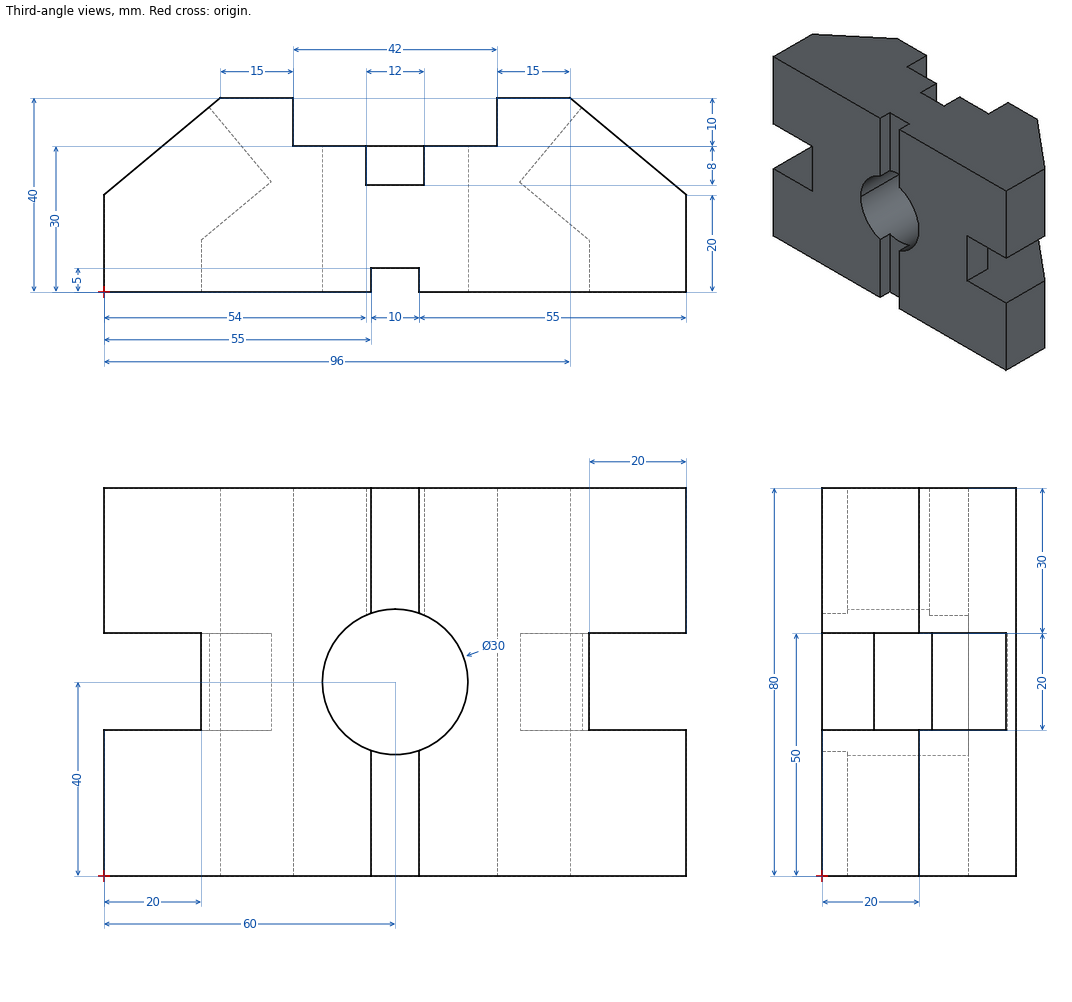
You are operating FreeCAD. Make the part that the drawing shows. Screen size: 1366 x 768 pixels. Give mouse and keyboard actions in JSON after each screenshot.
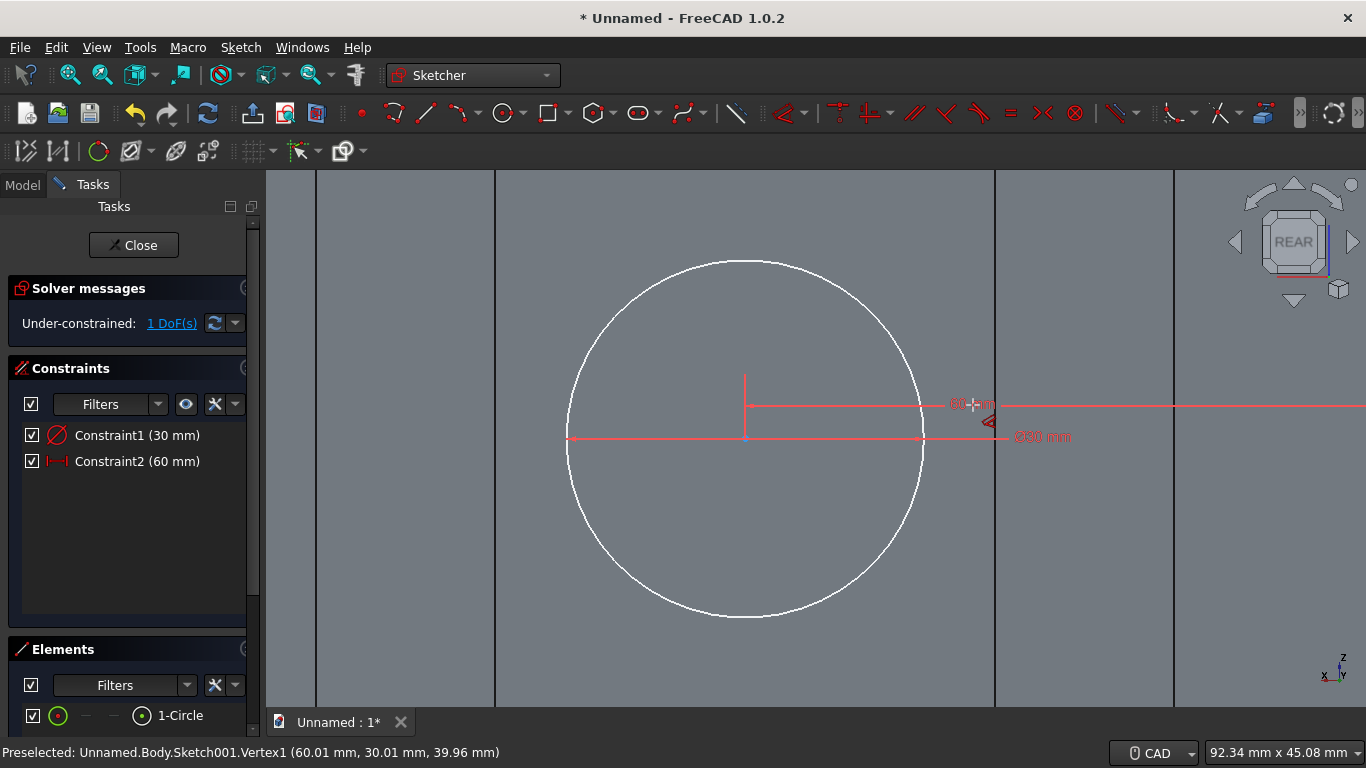
{"action": "left_click", "coordinate": [745, 439]}
{"action": "left_click", "coordinate": [711, 559]}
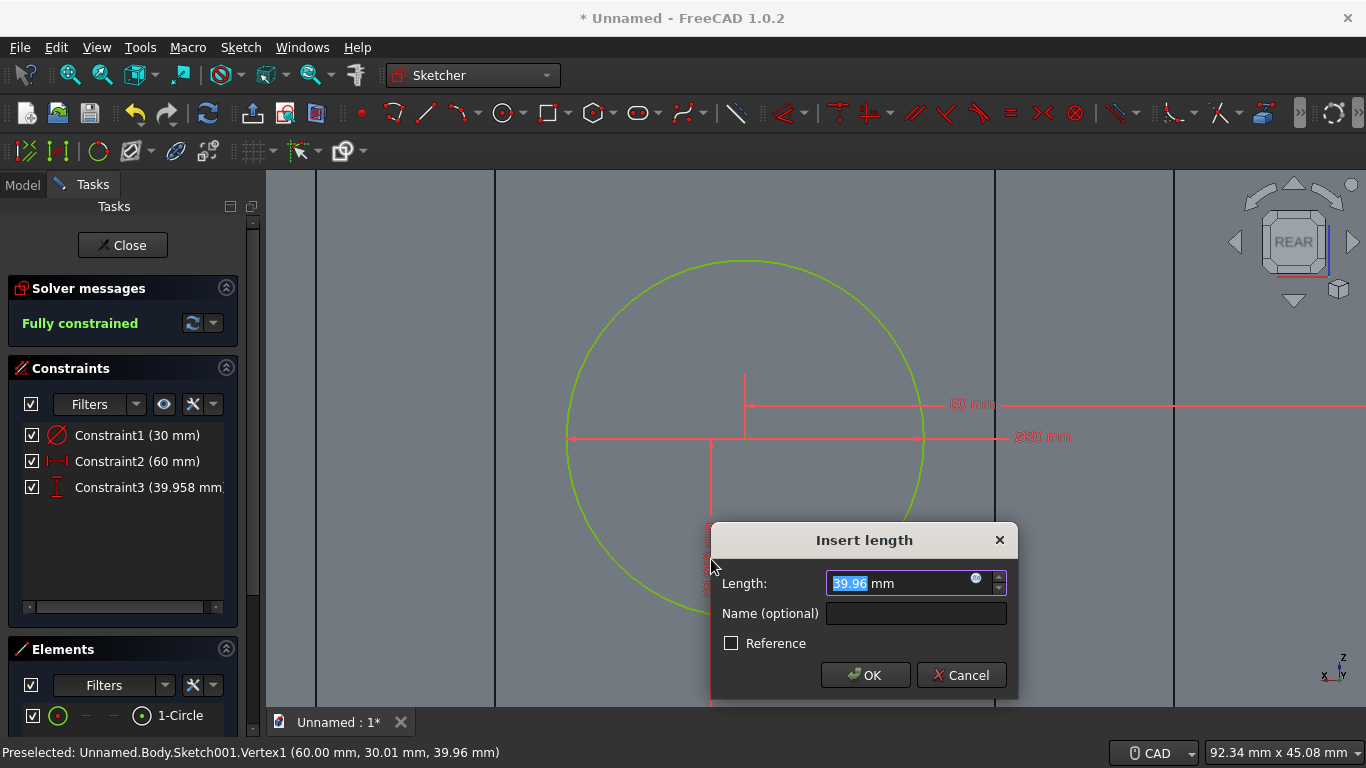
{"action": "type", "text": "40"}
{"action": "key", "text": "Return"}
{"action": "key", "text": "Escape"}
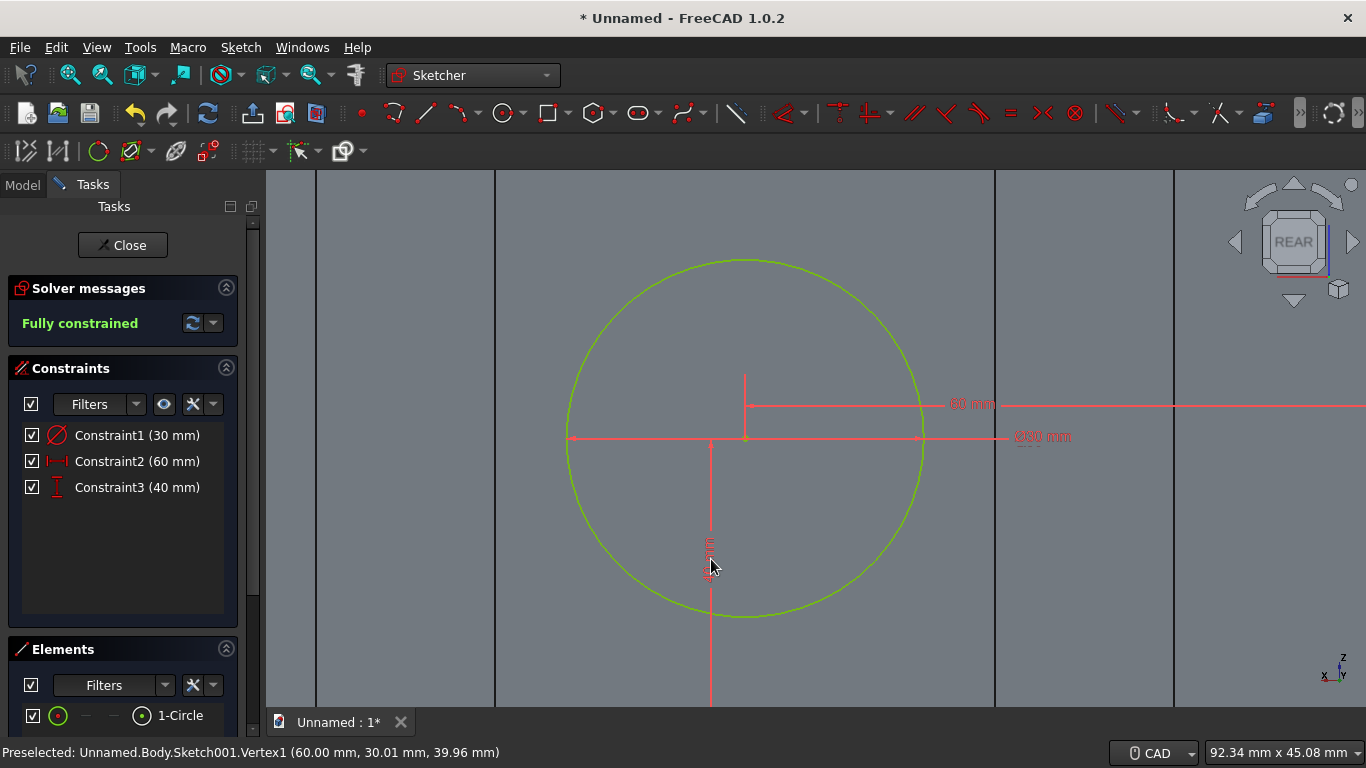
{"action": "left_click", "coordinate": [123, 245]}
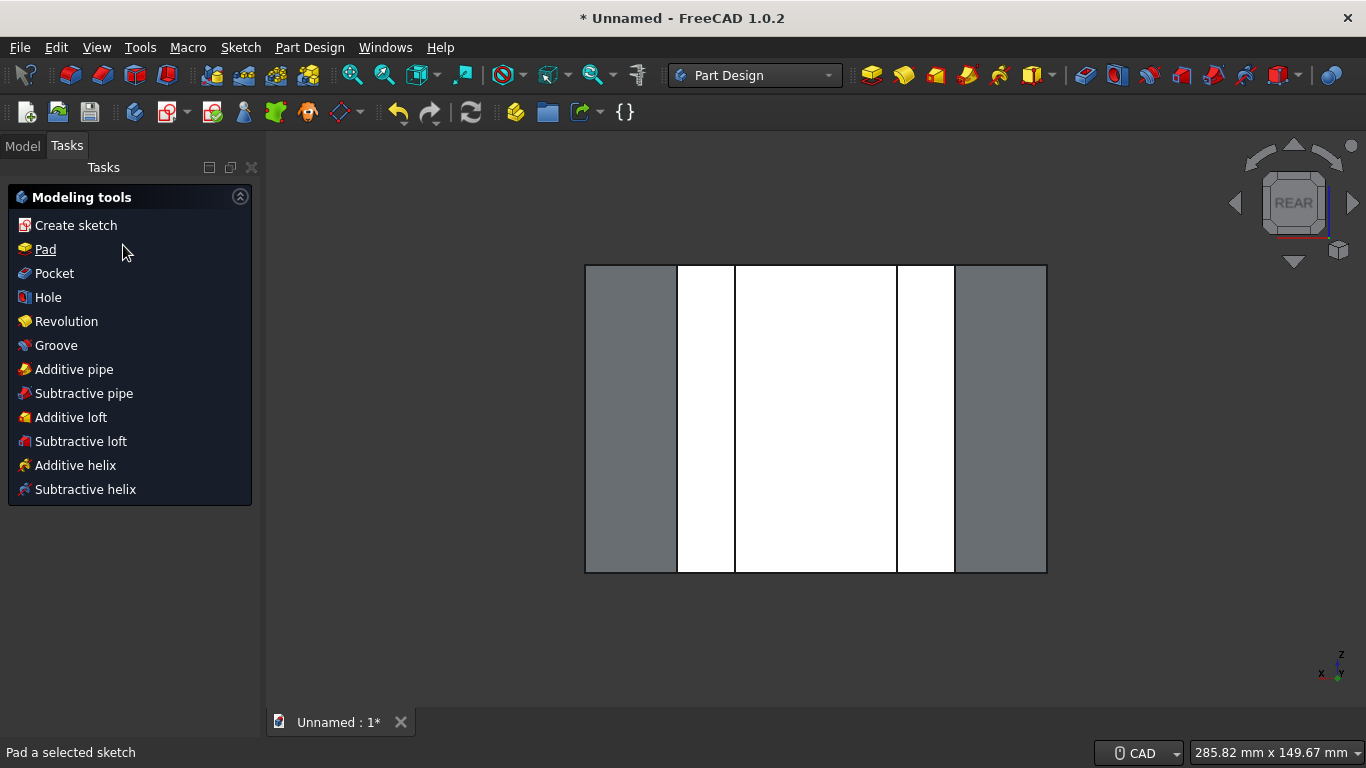
{"action": "left_click", "coordinate": [1086, 76]}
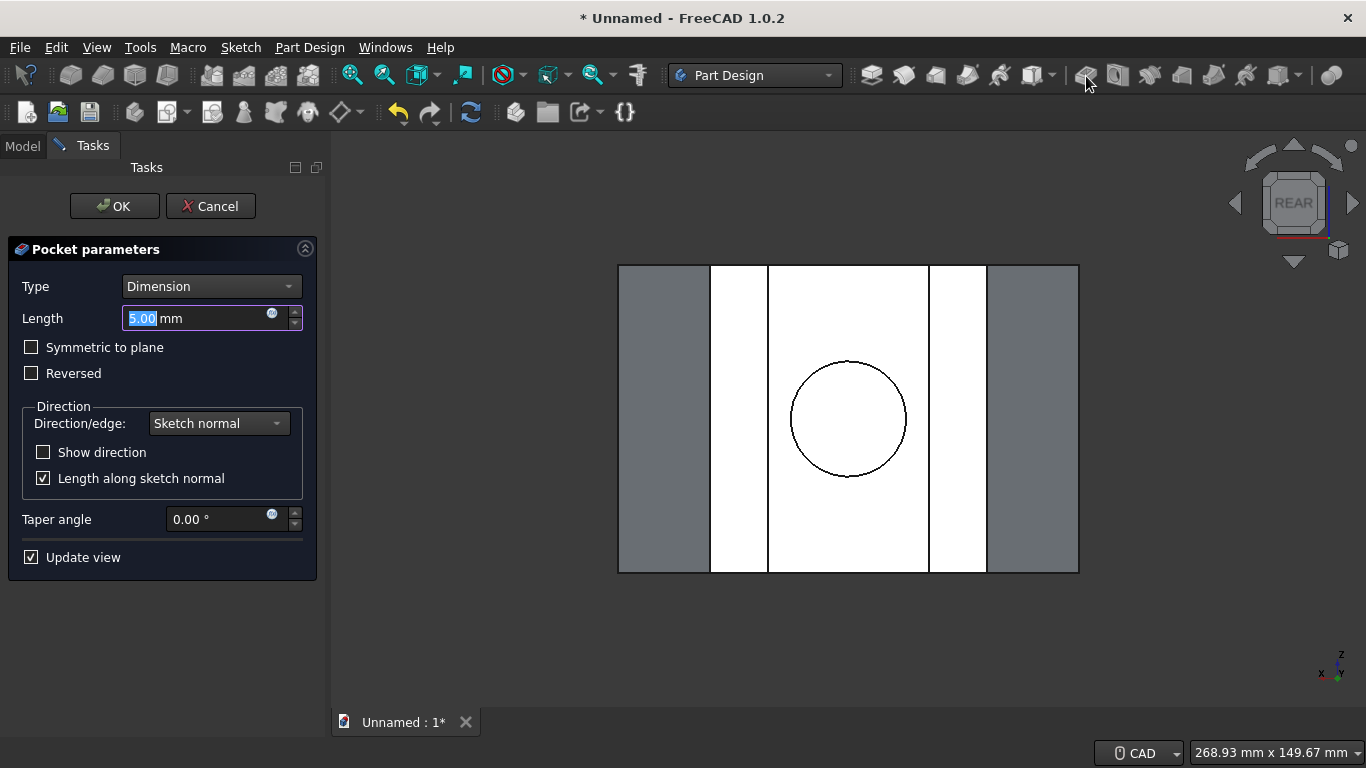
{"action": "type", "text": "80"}
{"action": "key", "text": "Tab"}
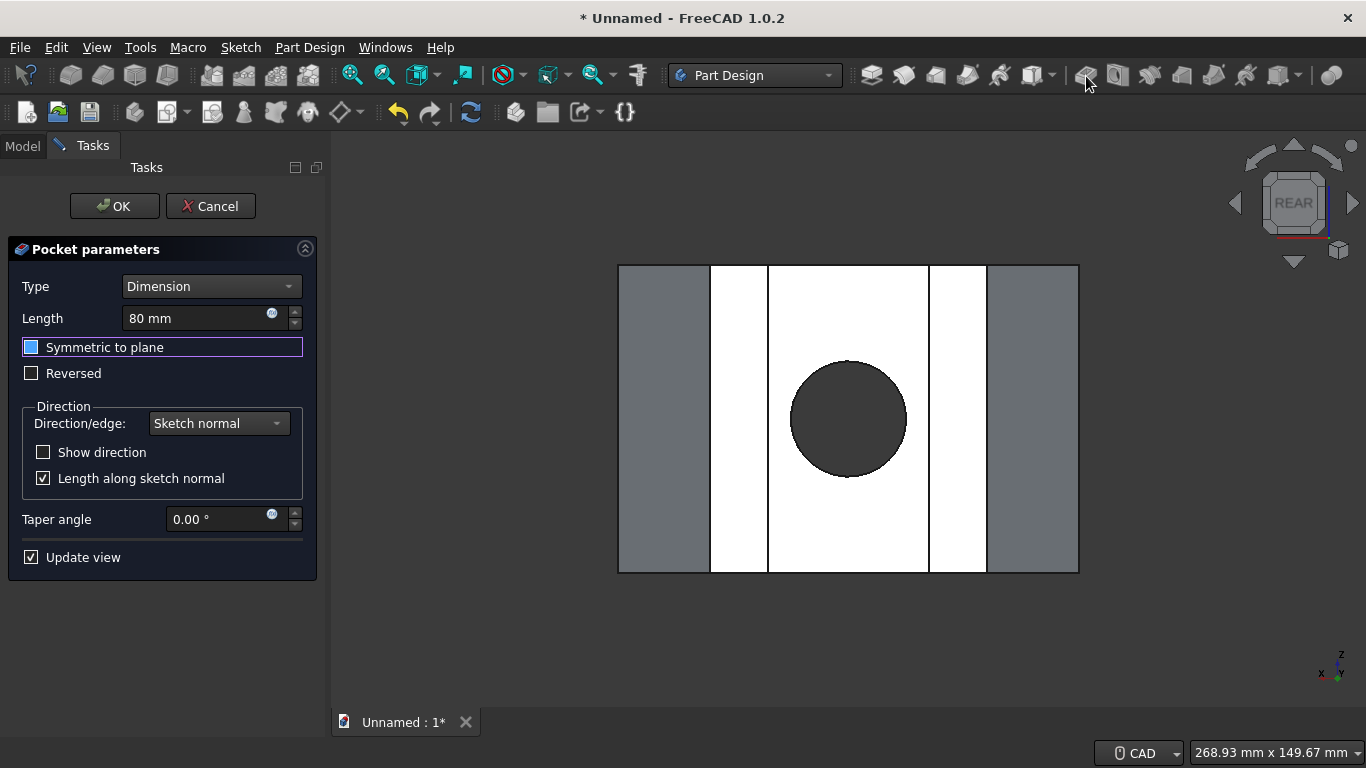
{"action": "left_click", "coordinate": [115, 206]}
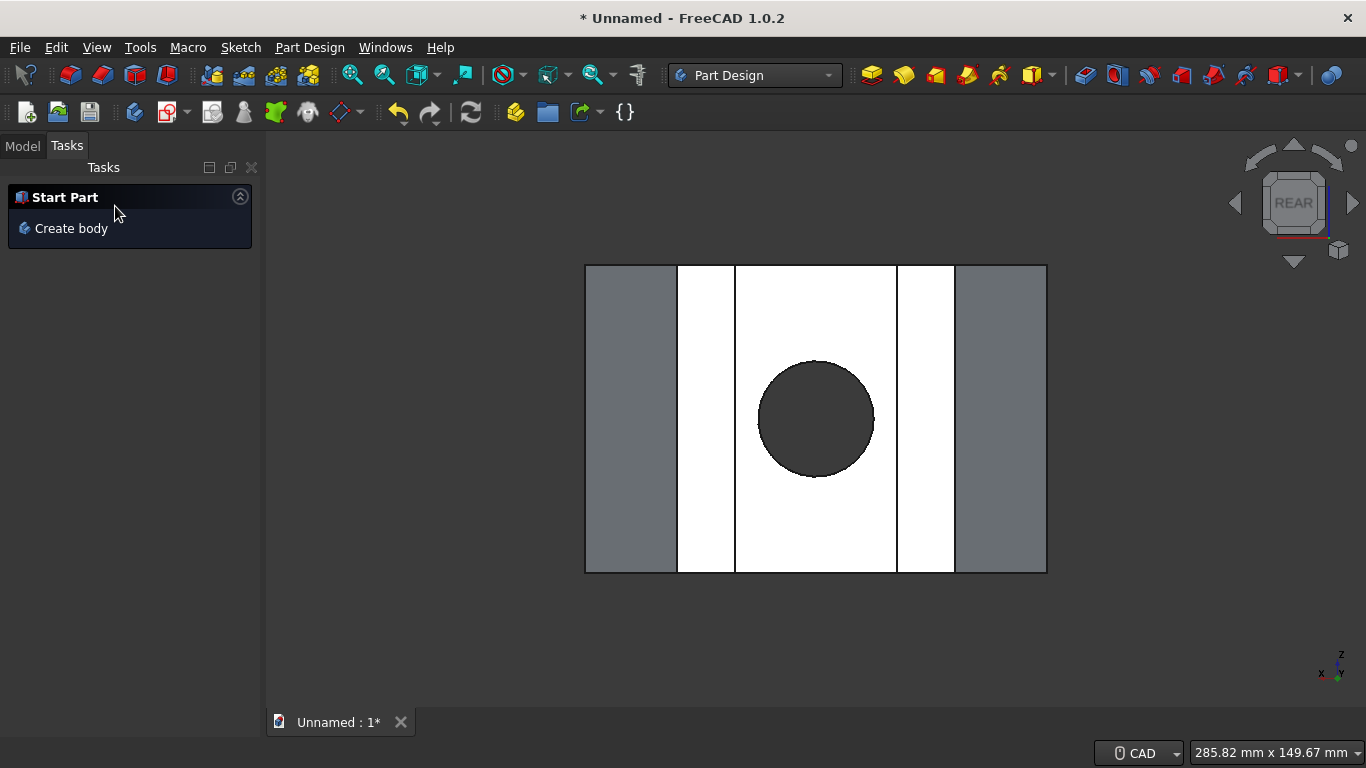
{"action": "key", "text": "0"}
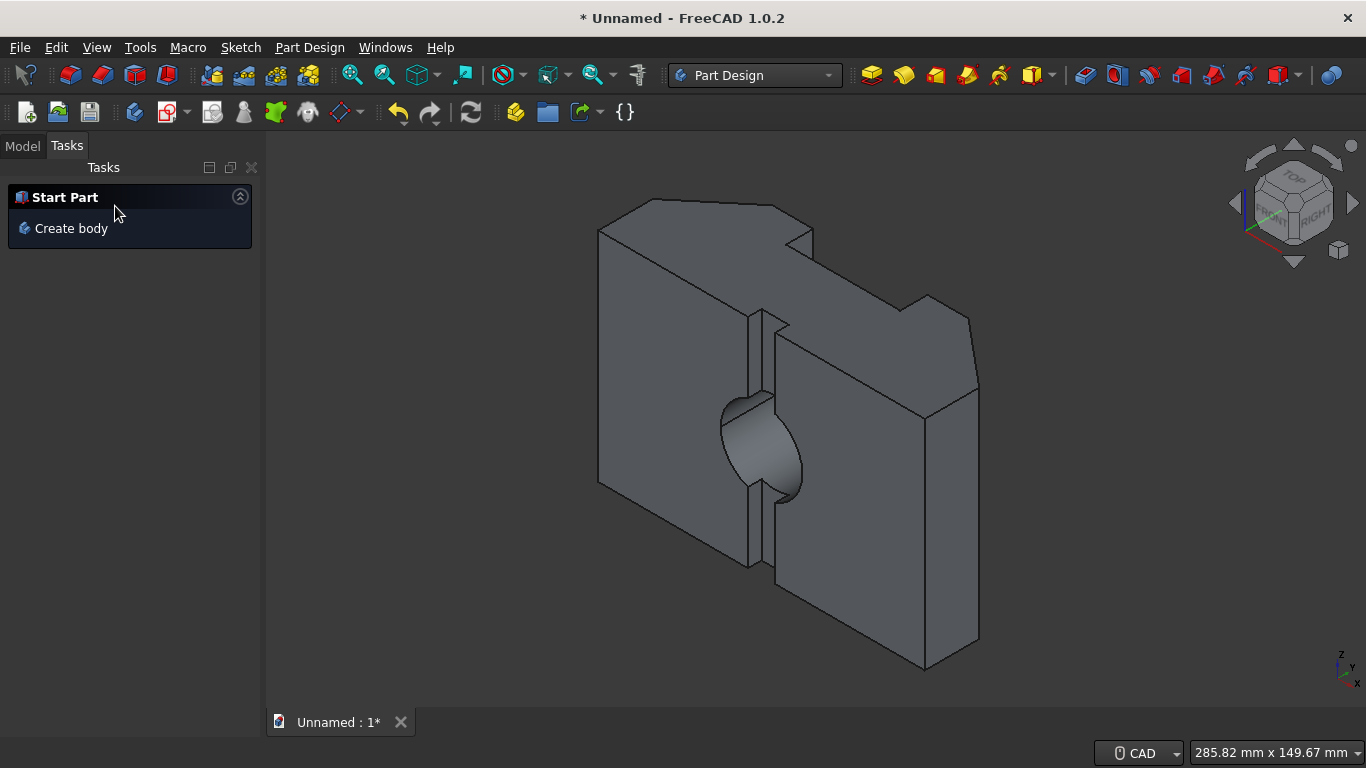
{"action": "left_click", "coordinate": [909, 346]}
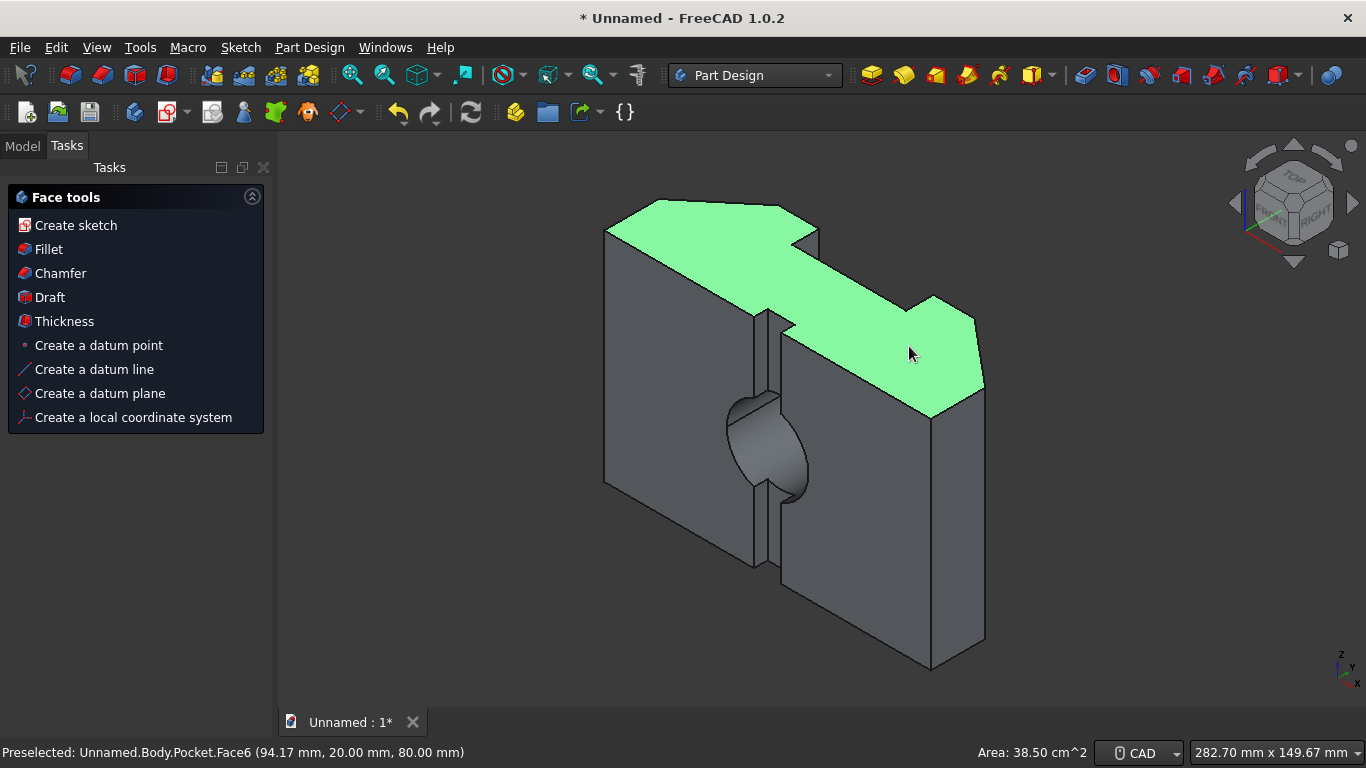
{"action": "left_click", "coordinate": [168, 112]}